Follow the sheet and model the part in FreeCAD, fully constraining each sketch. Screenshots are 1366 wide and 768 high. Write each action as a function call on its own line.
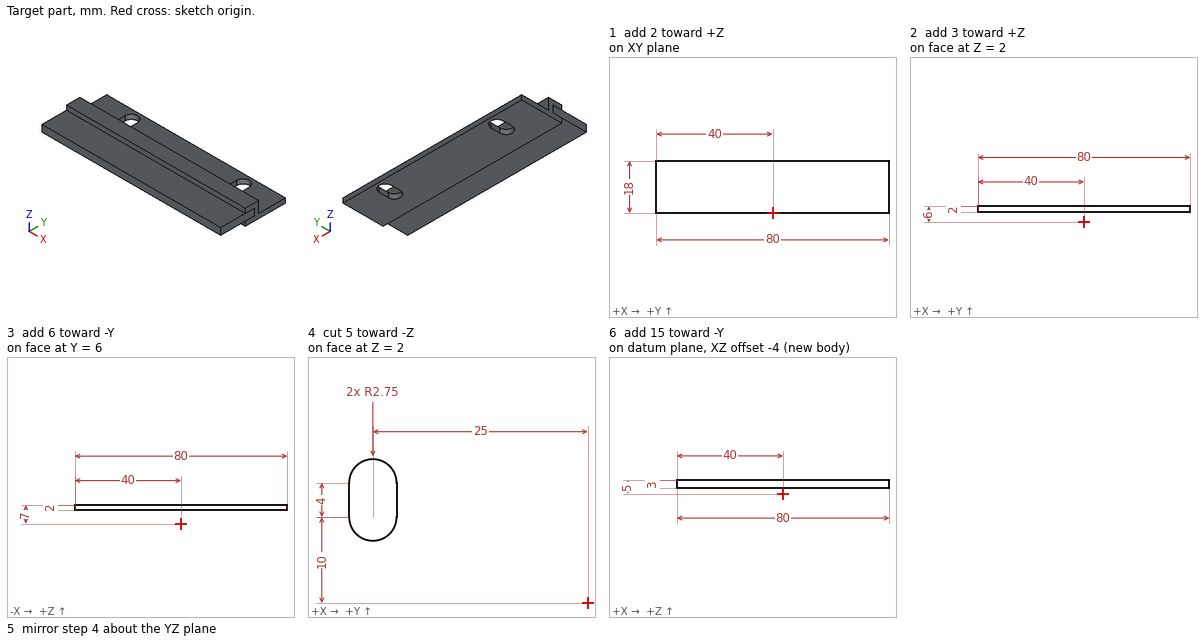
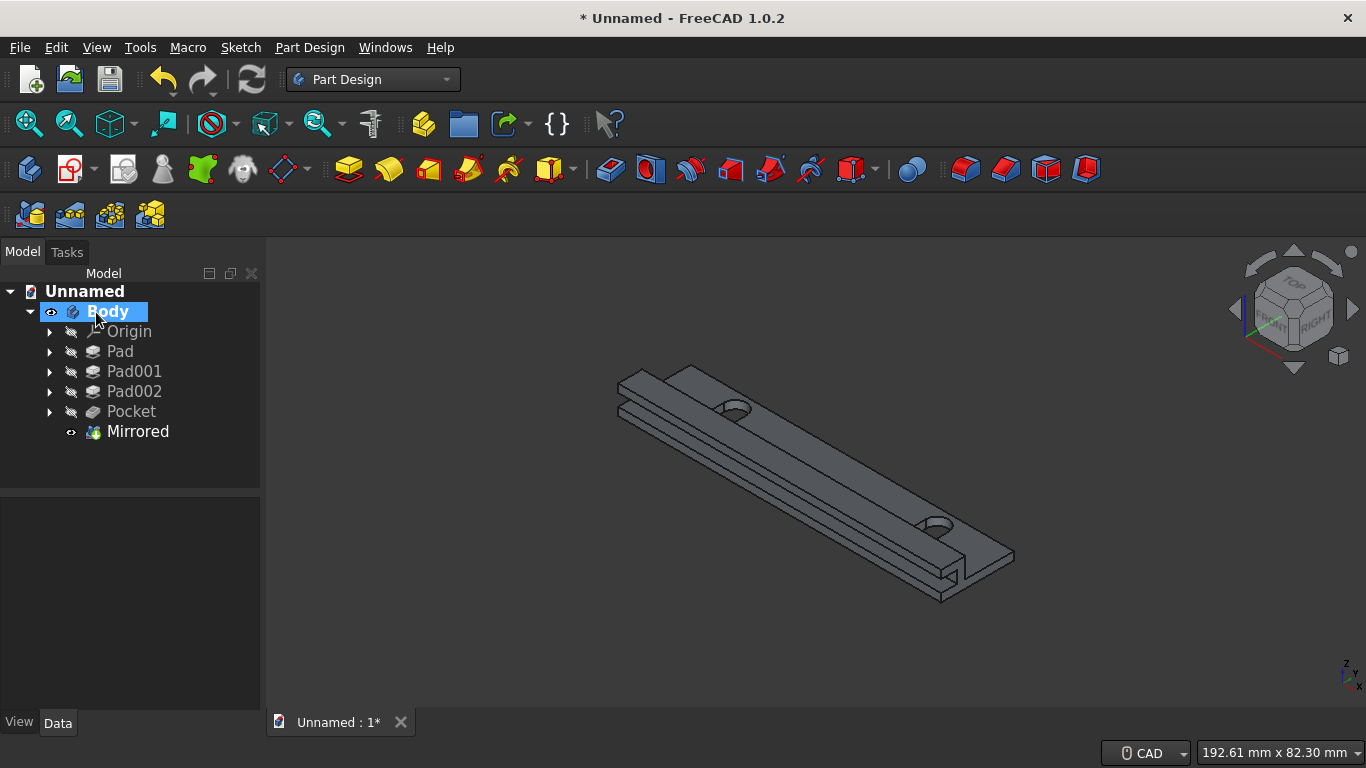
click(30, 170)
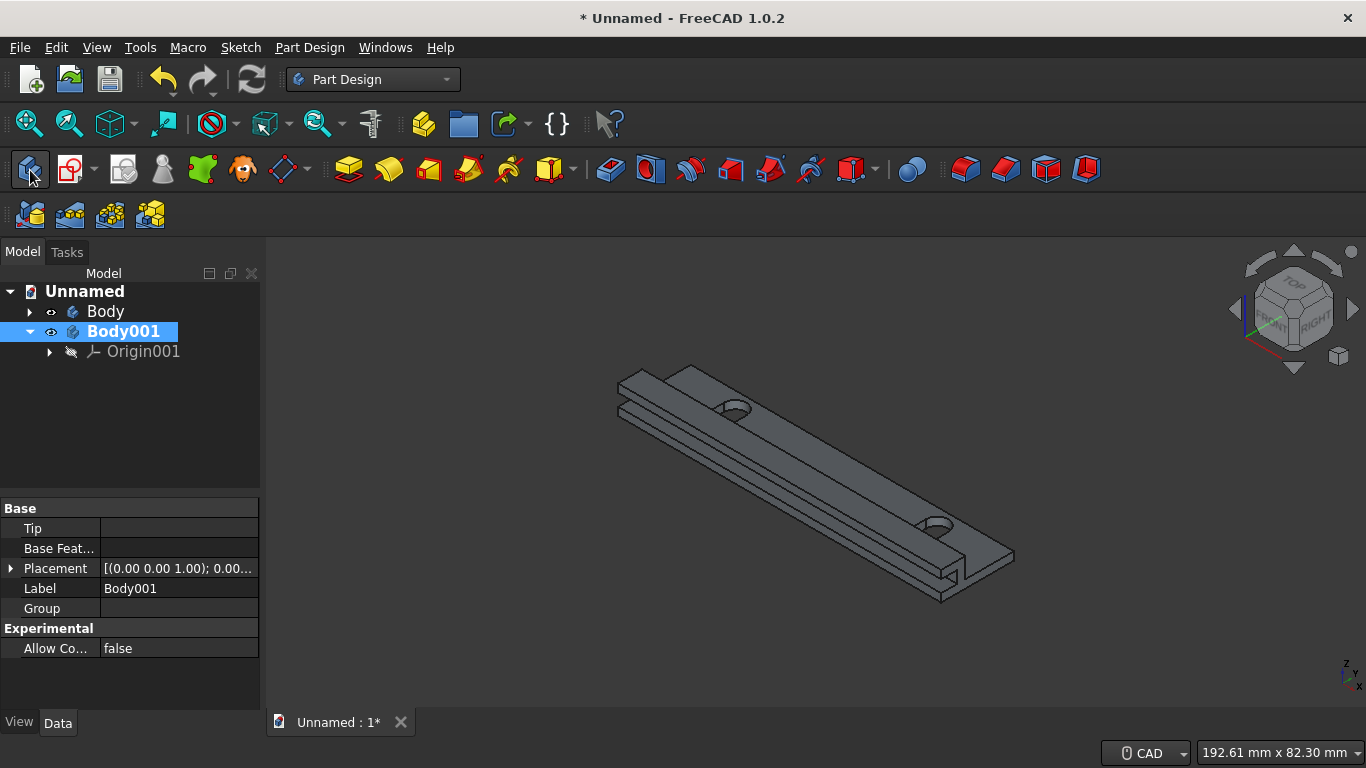
click(50, 352)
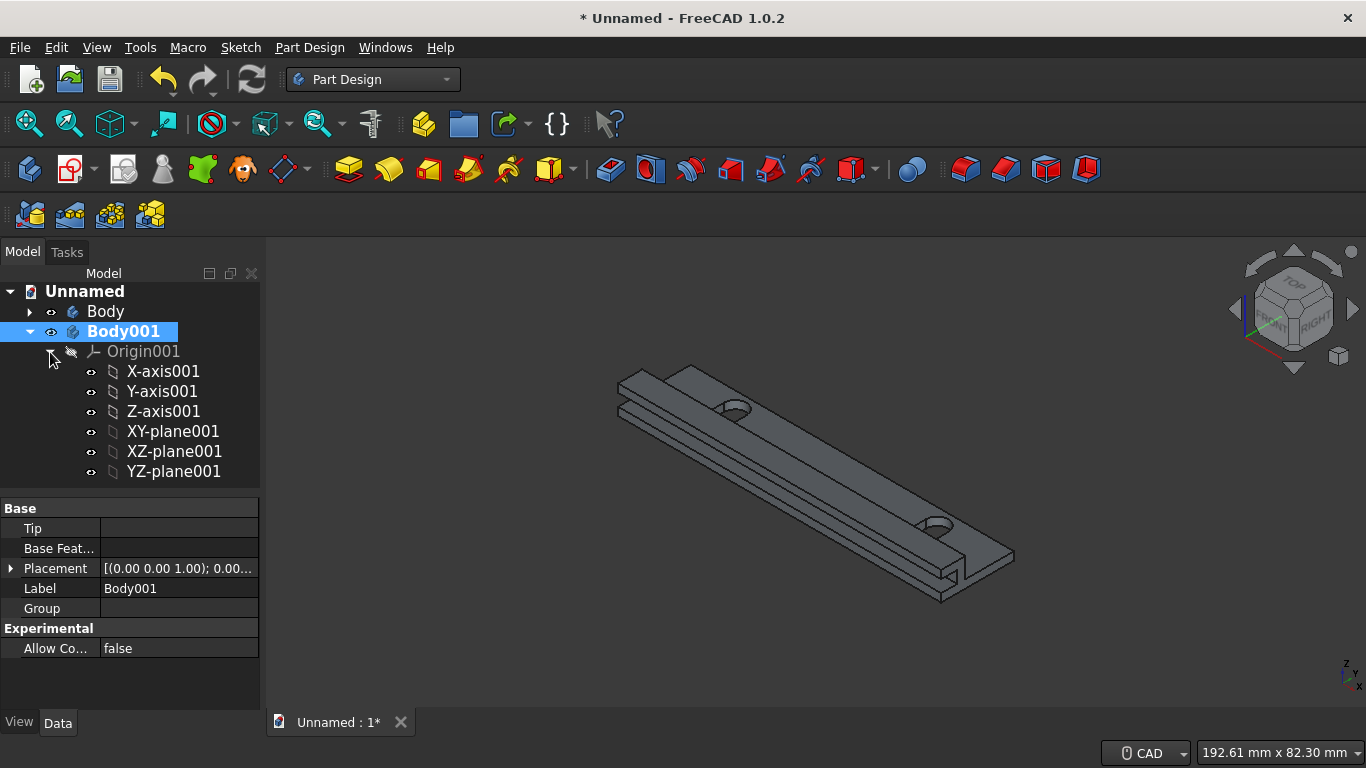
click(136, 452)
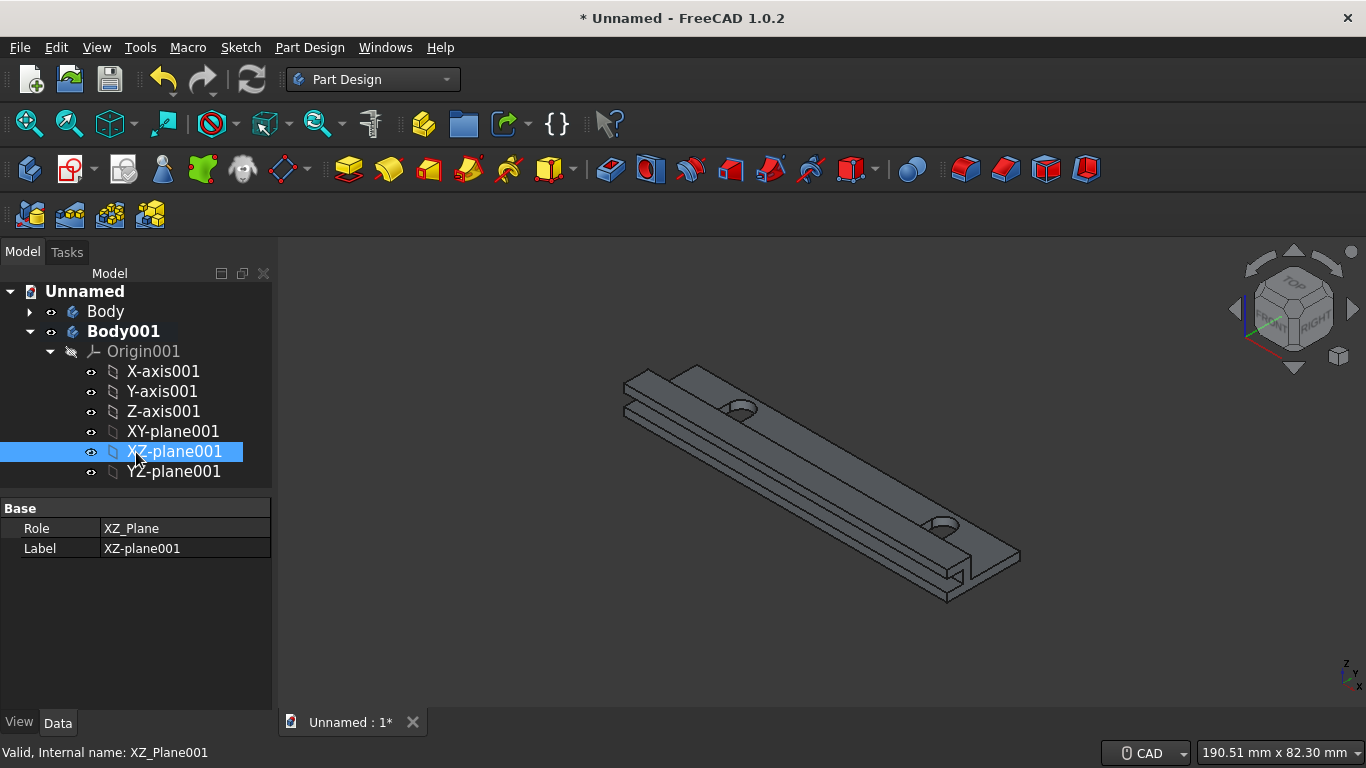
click(284, 170)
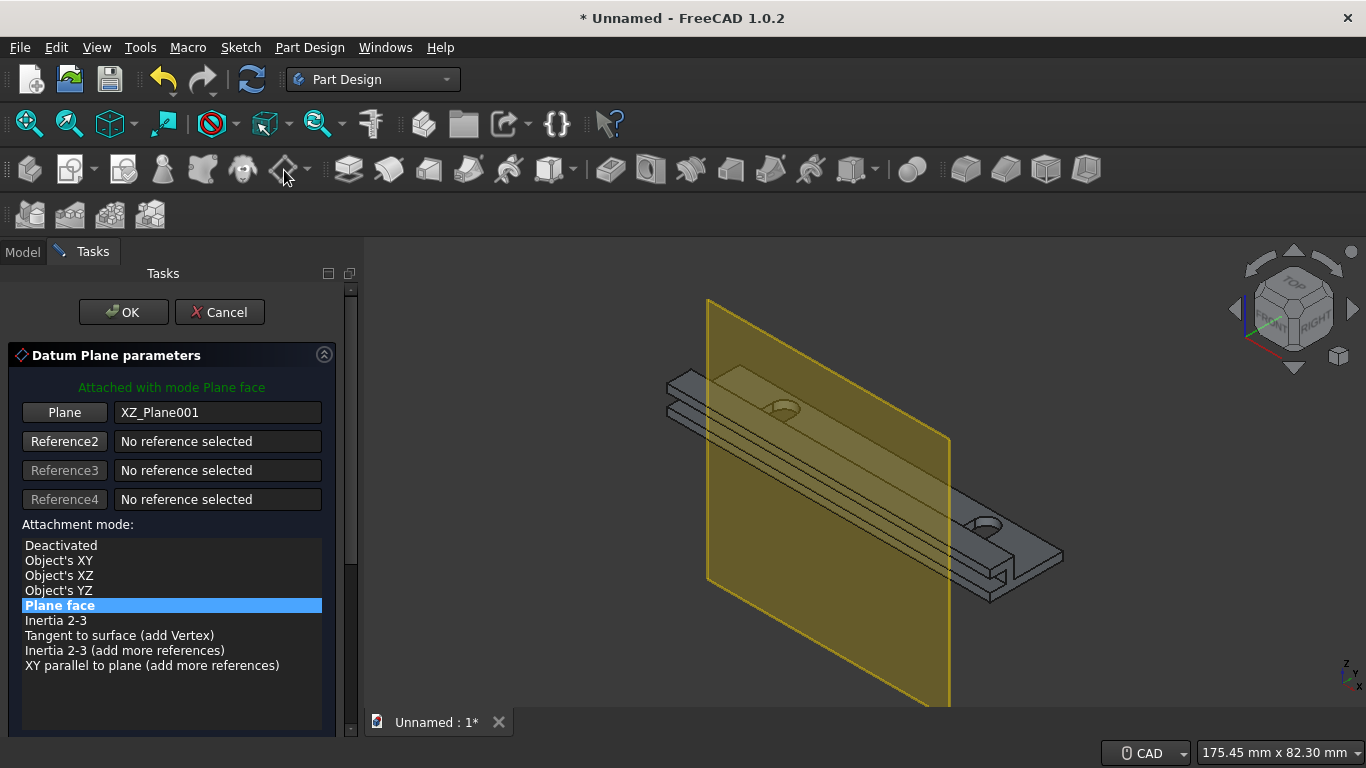
scroll(351, 510, down, 3)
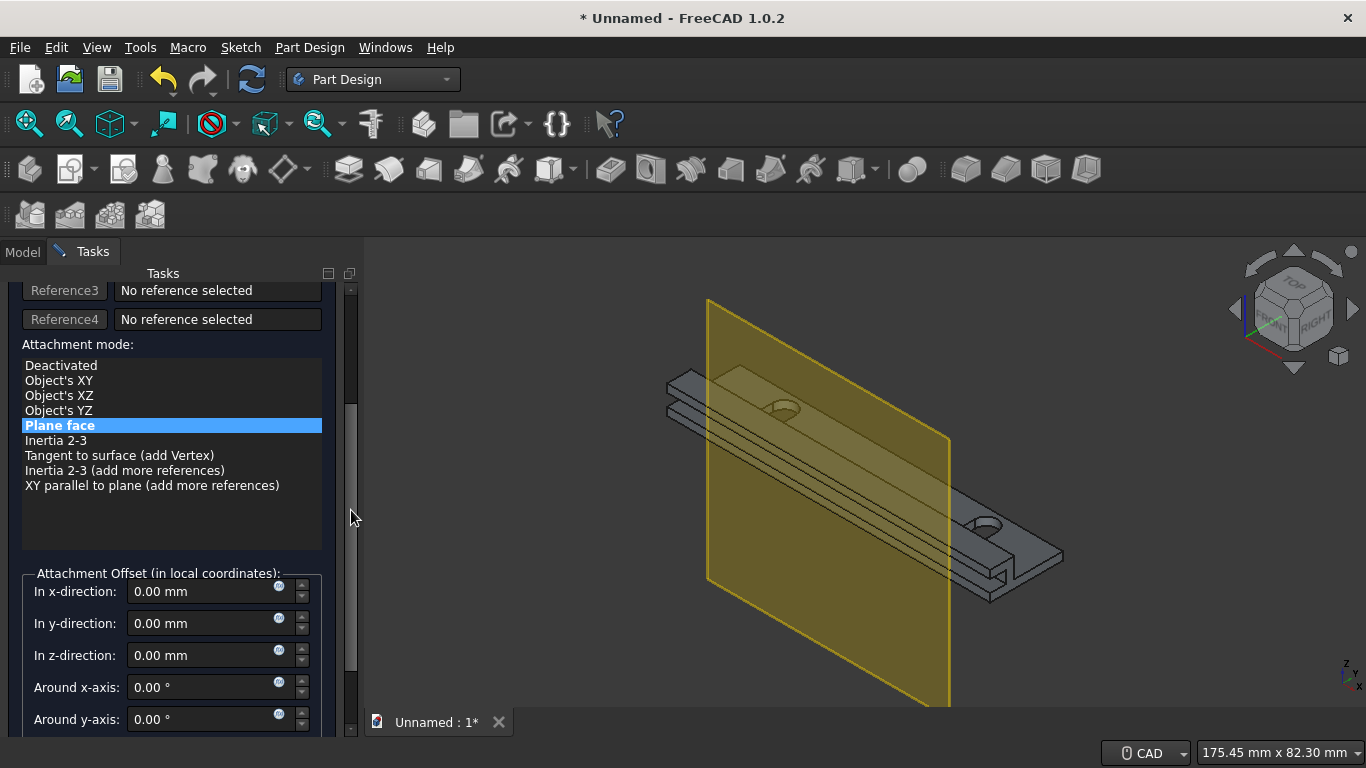
triple_click(210, 655)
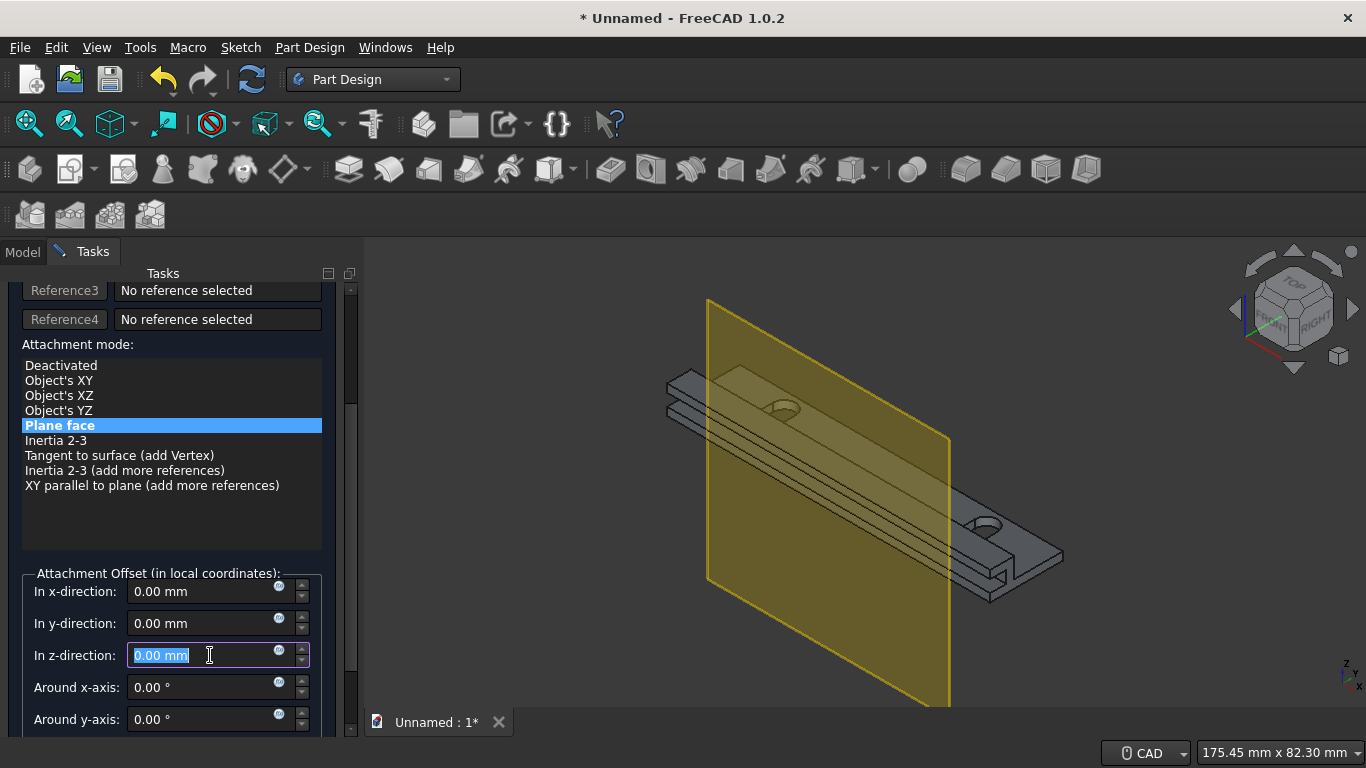
text(-4)
key(Tab)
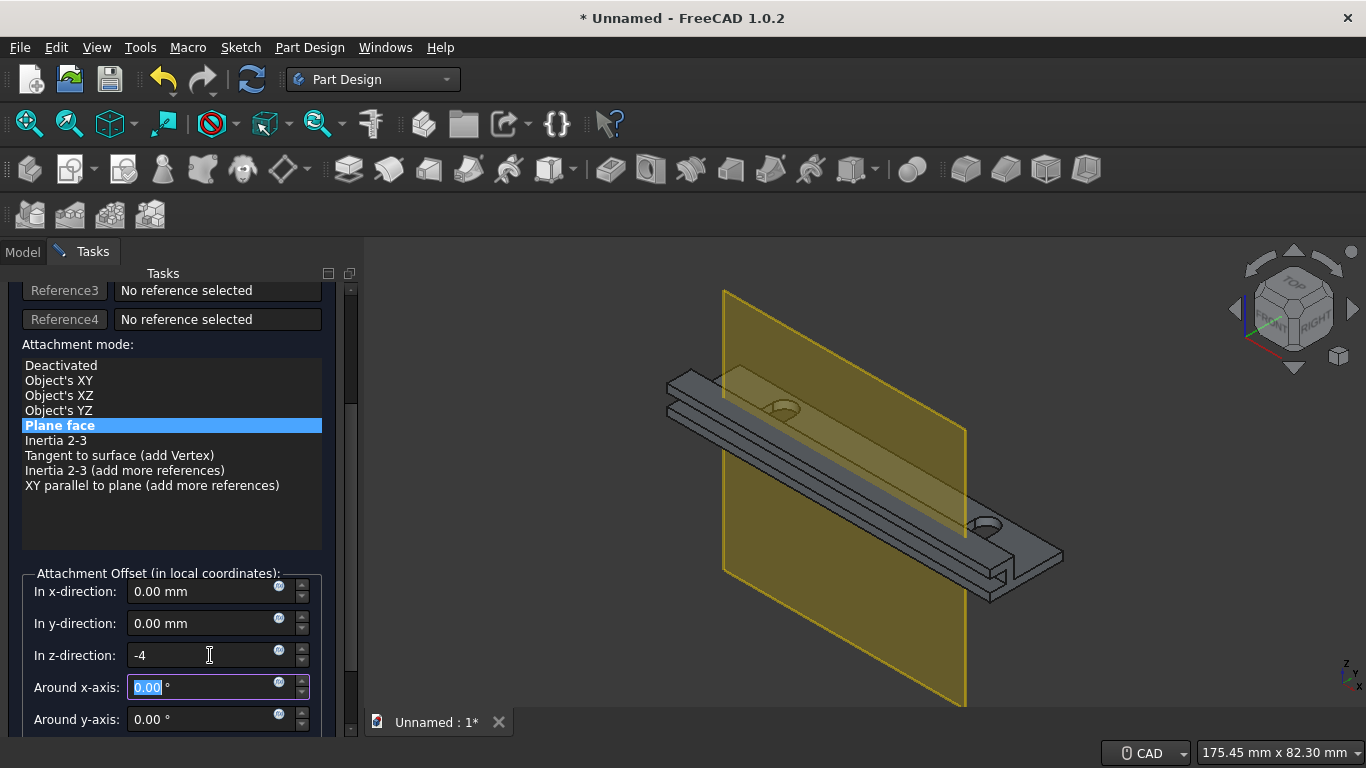
scroll(351, 510, up, 4)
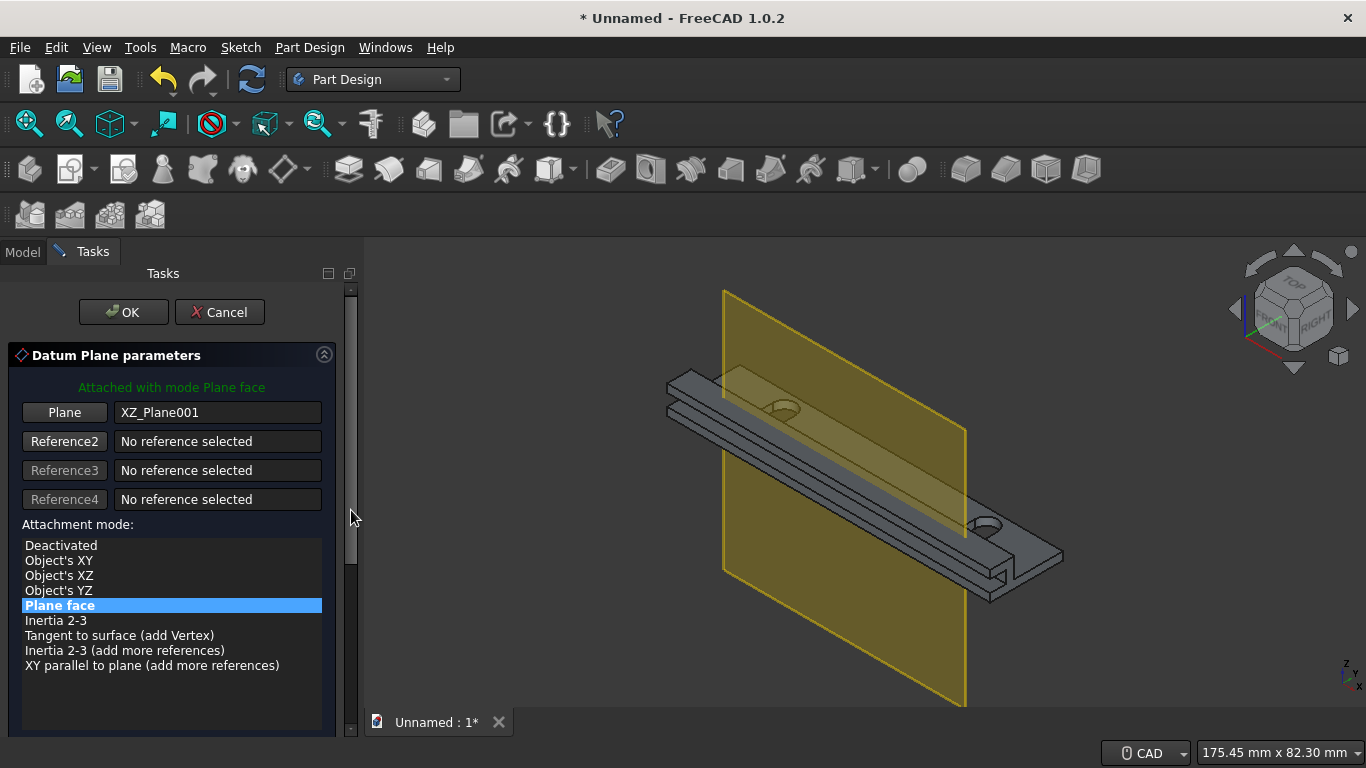
click(124, 312)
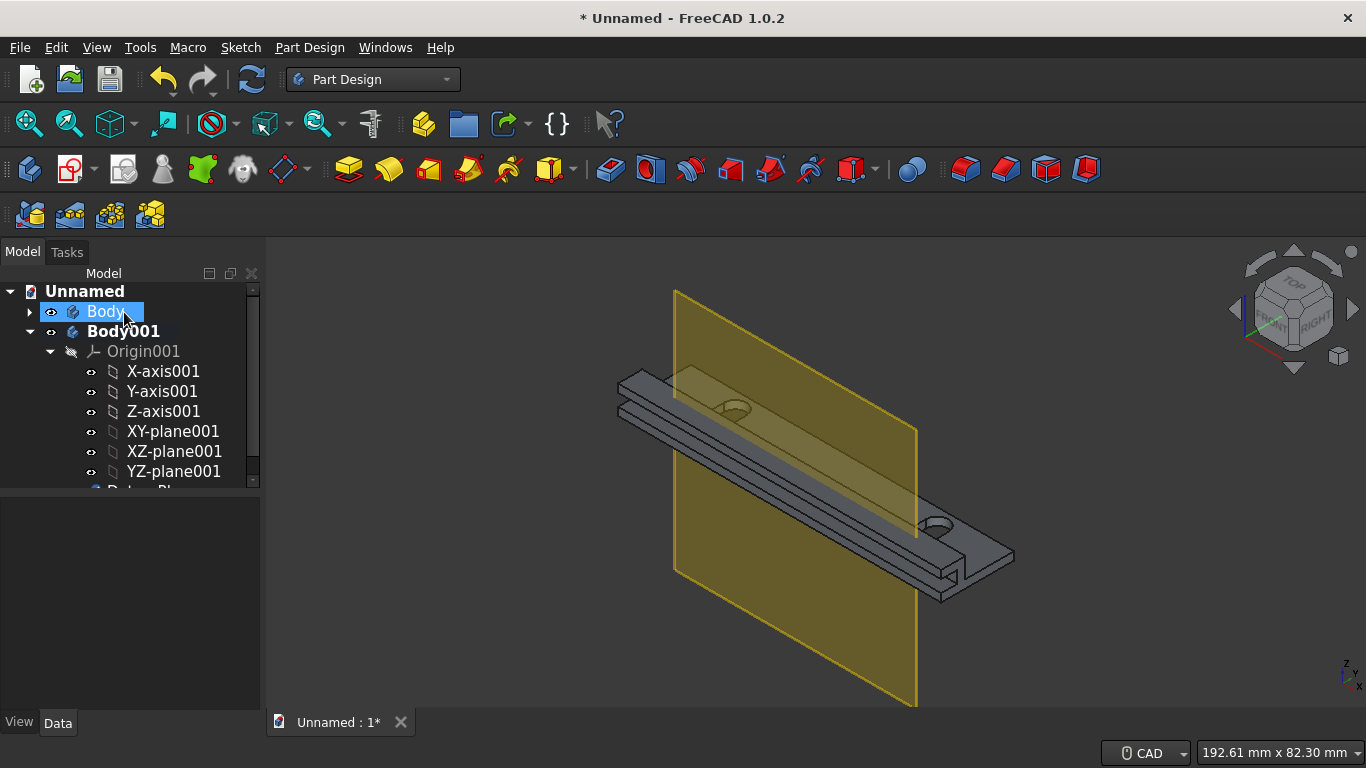
scroll(100, 387, down, 3)